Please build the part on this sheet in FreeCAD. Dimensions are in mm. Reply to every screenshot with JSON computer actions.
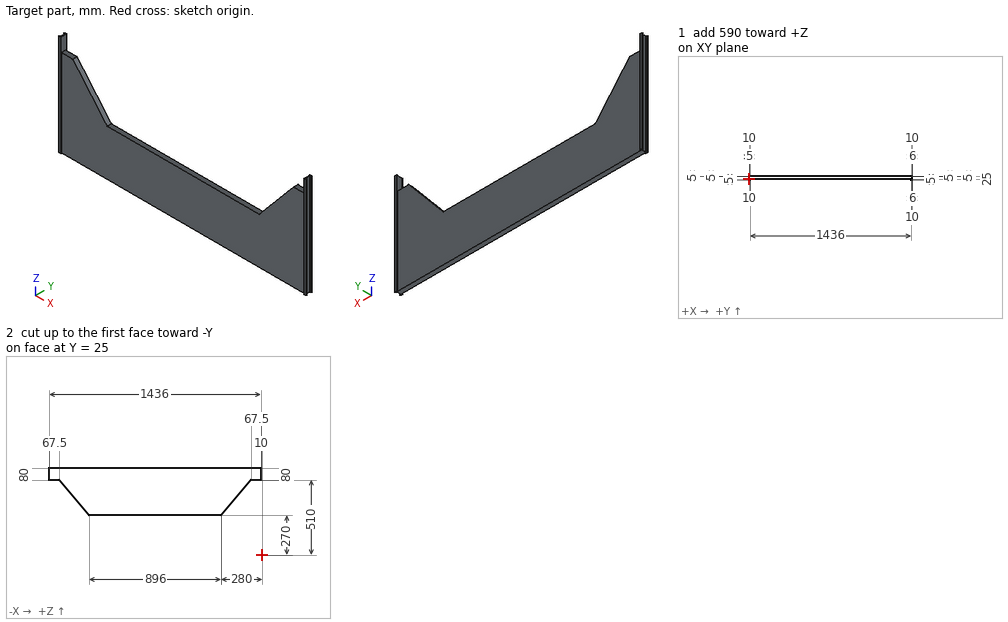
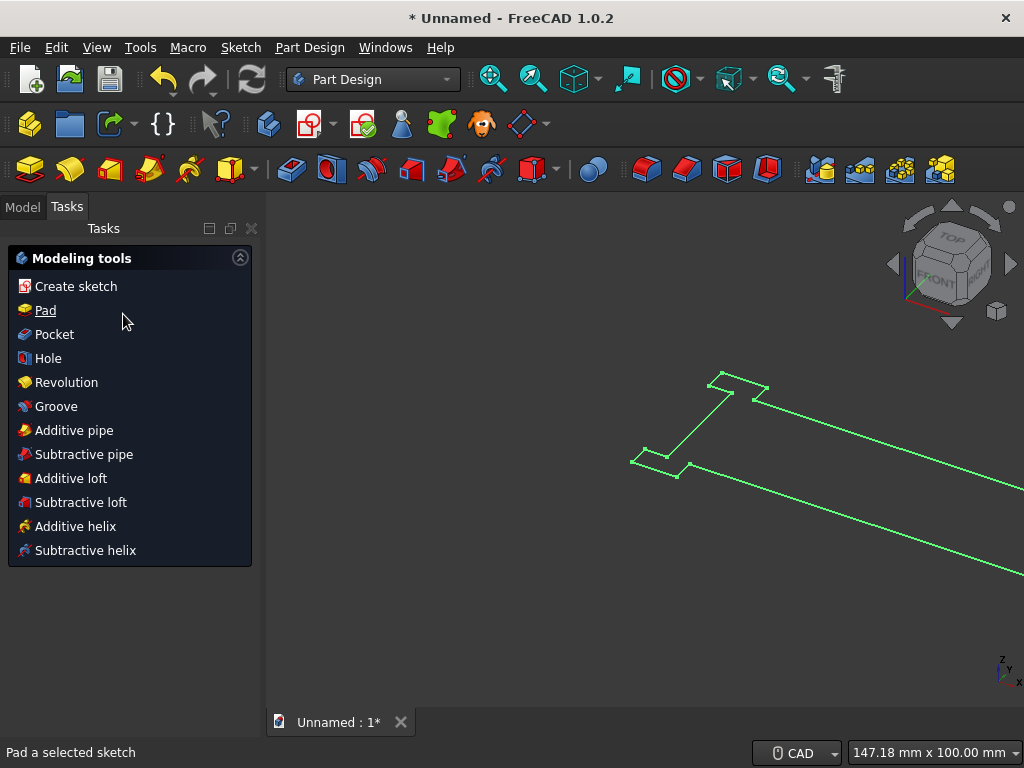
{"action": "left_click", "coordinate": [30, 170]}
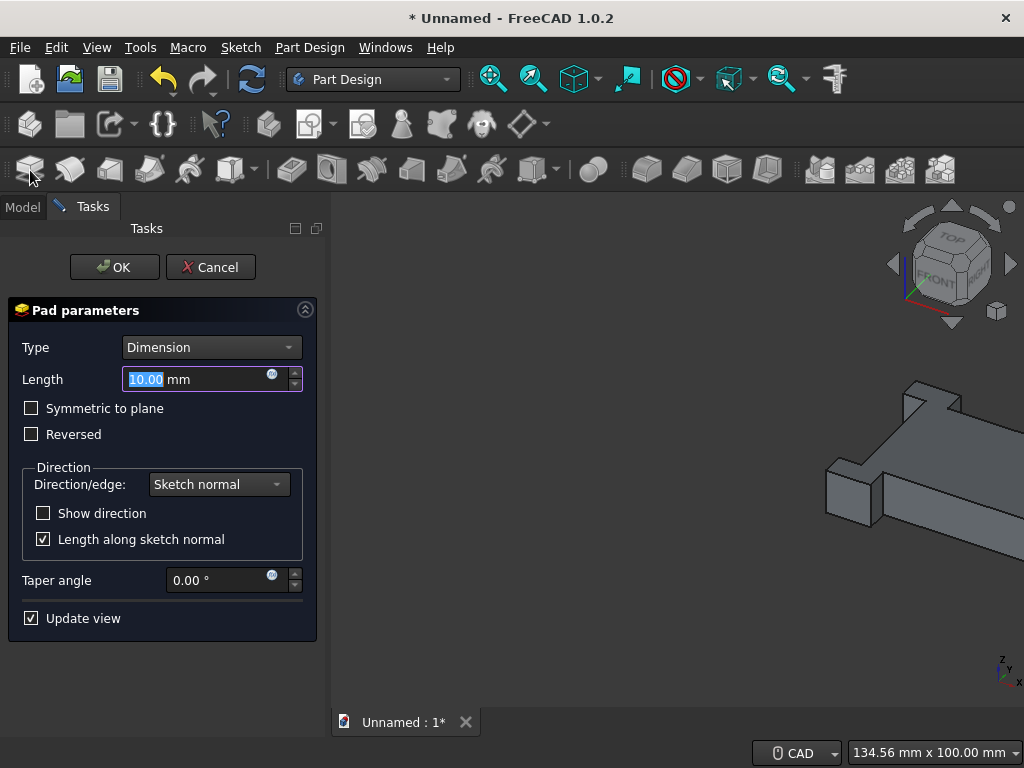
{"action": "type", "text": "590"}
{"action": "key", "text": "Tab"}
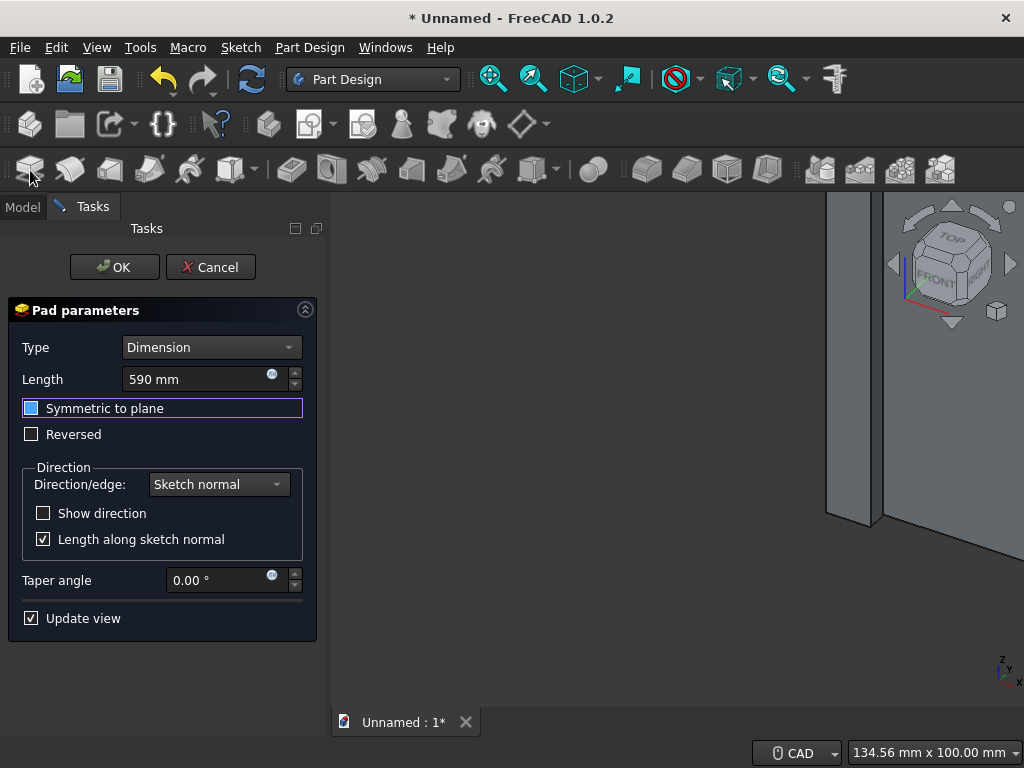
{"action": "left_click", "coordinate": [115, 267]}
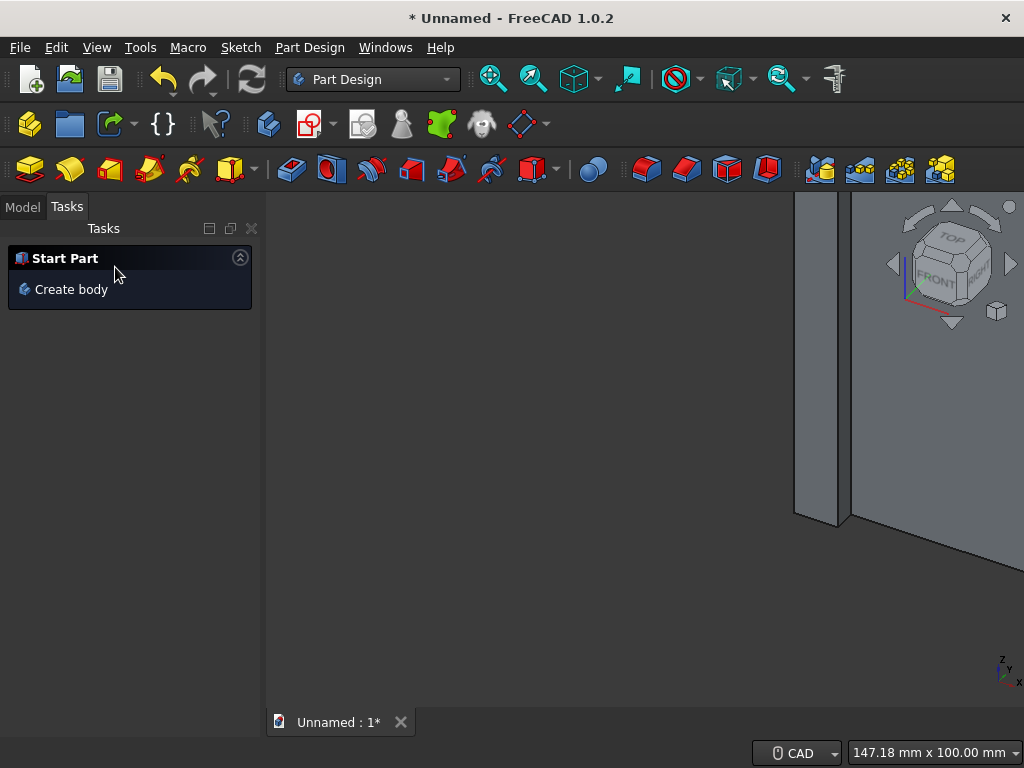
{"action": "left_click", "coordinate": [494, 80]}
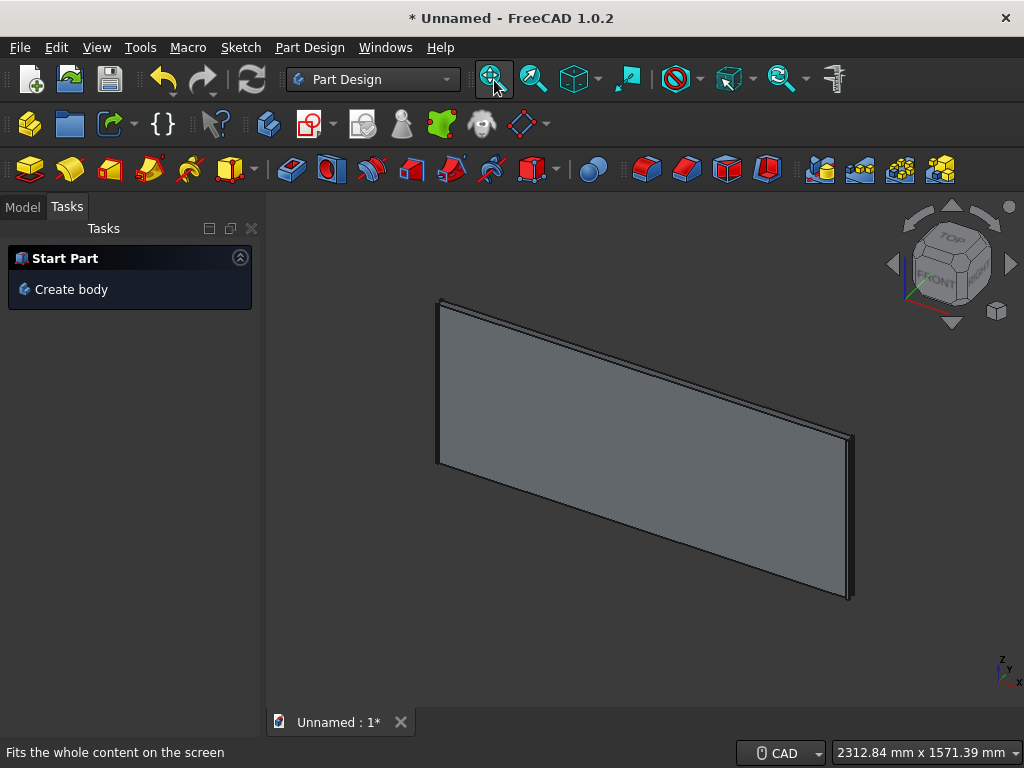
{"action": "key", "text": "4"}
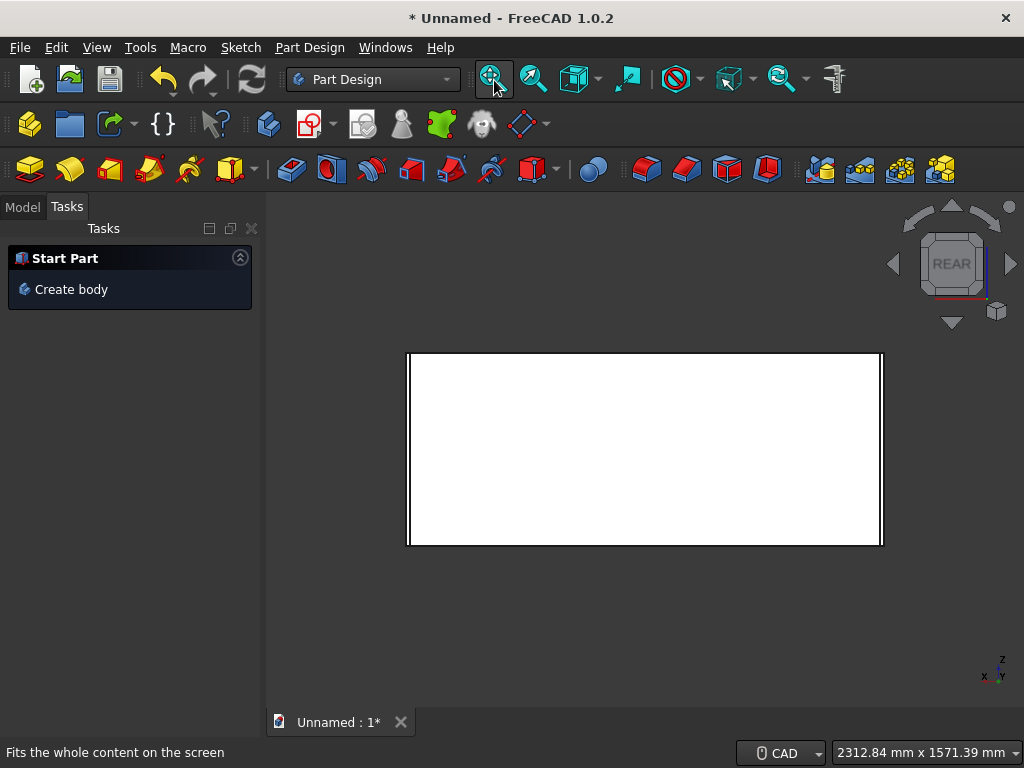
{"action": "left_click", "coordinate": [511, 448]}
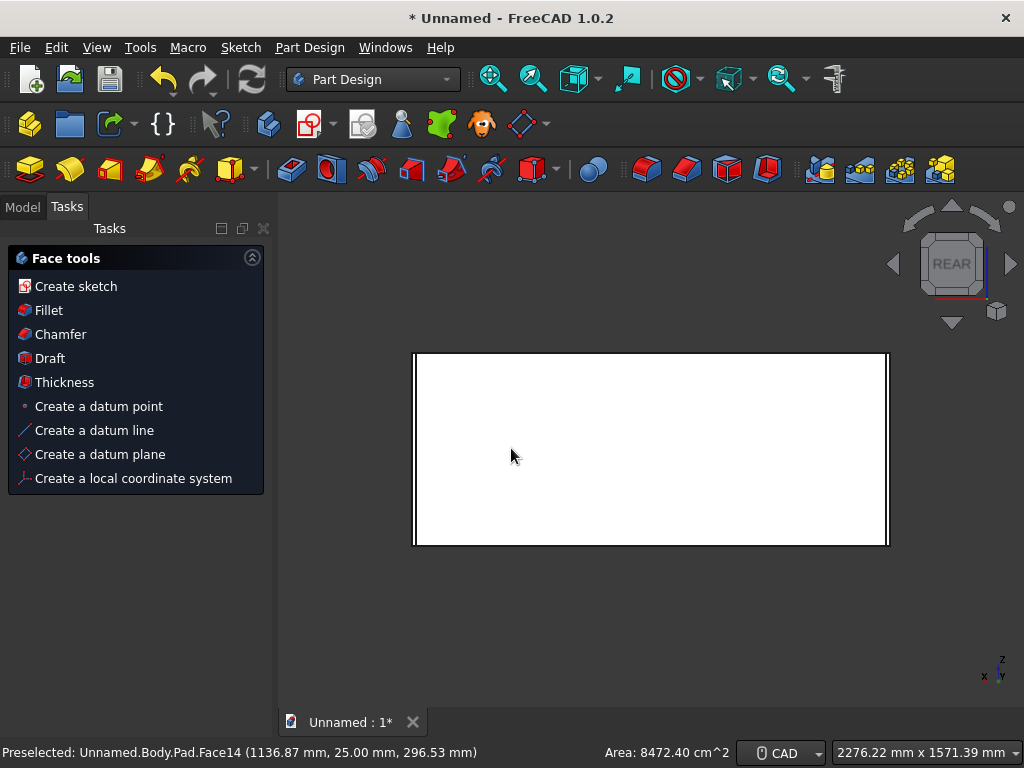
{"action": "left_click", "coordinate": [310, 124]}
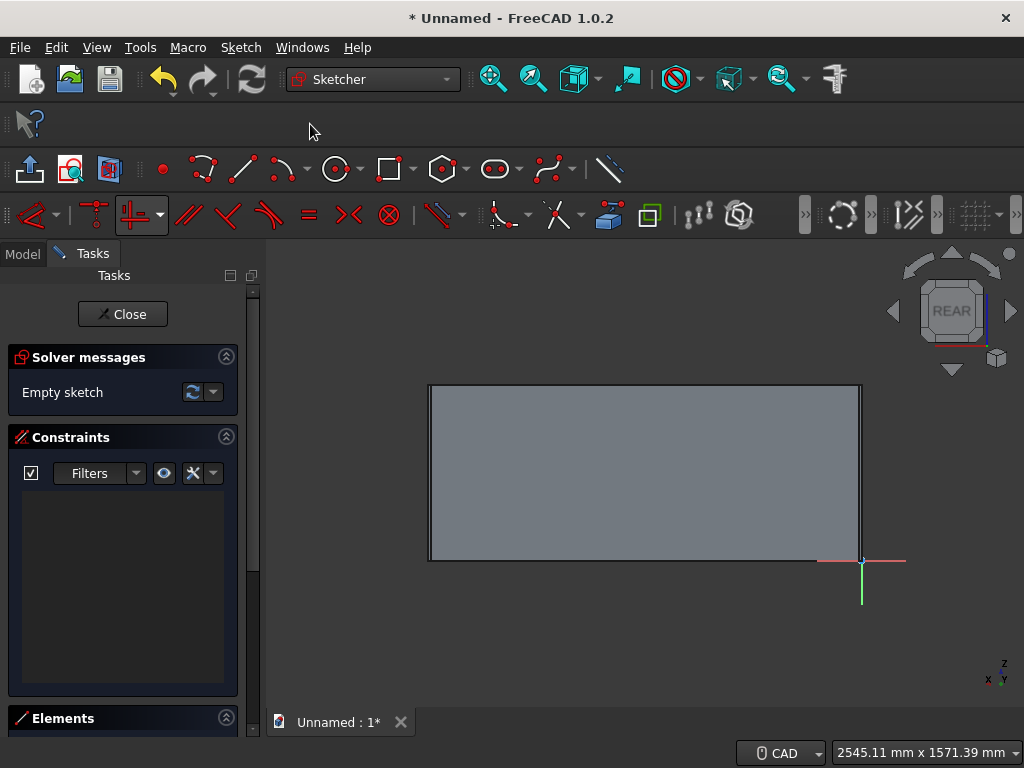
{"action": "key", "text": "q s"}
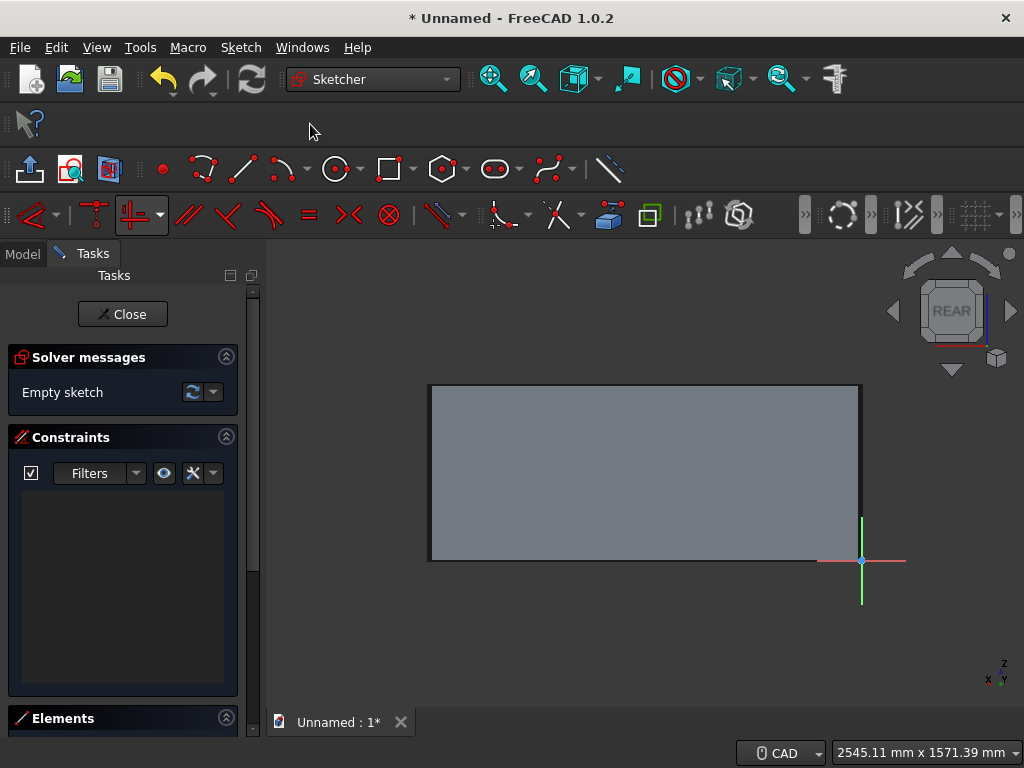
{"action": "scroll", "coordinate": [294, 473], "scroll_direction": "down", "scroll_amount": 1}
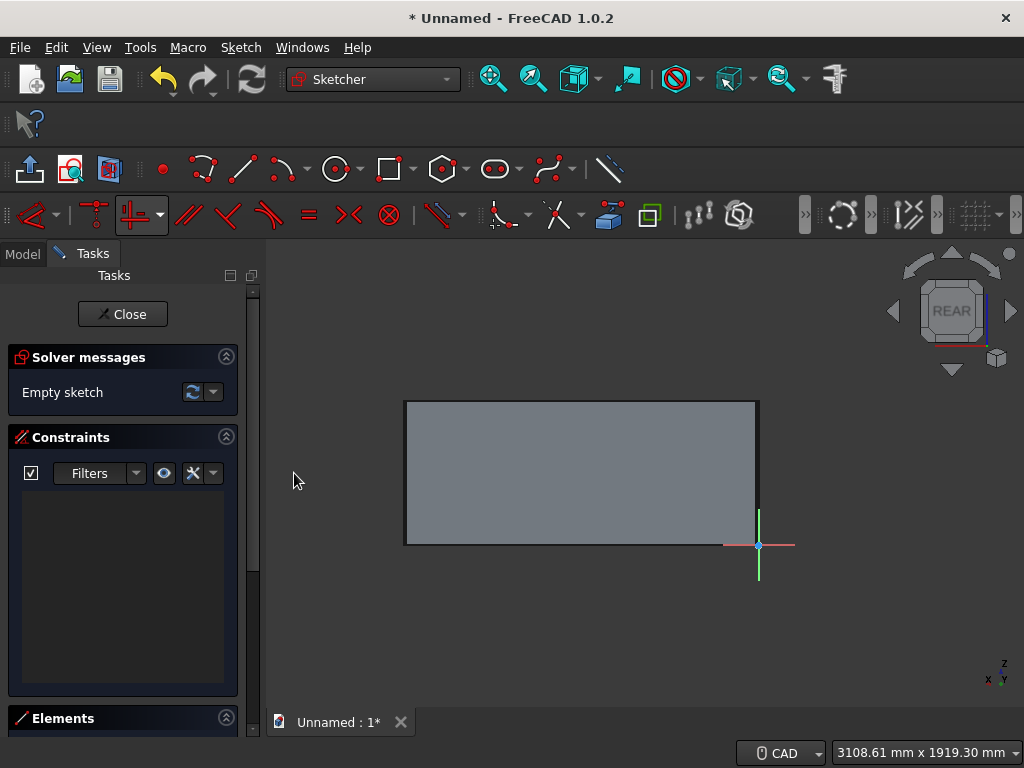
{"action": "key", "text": "g m"}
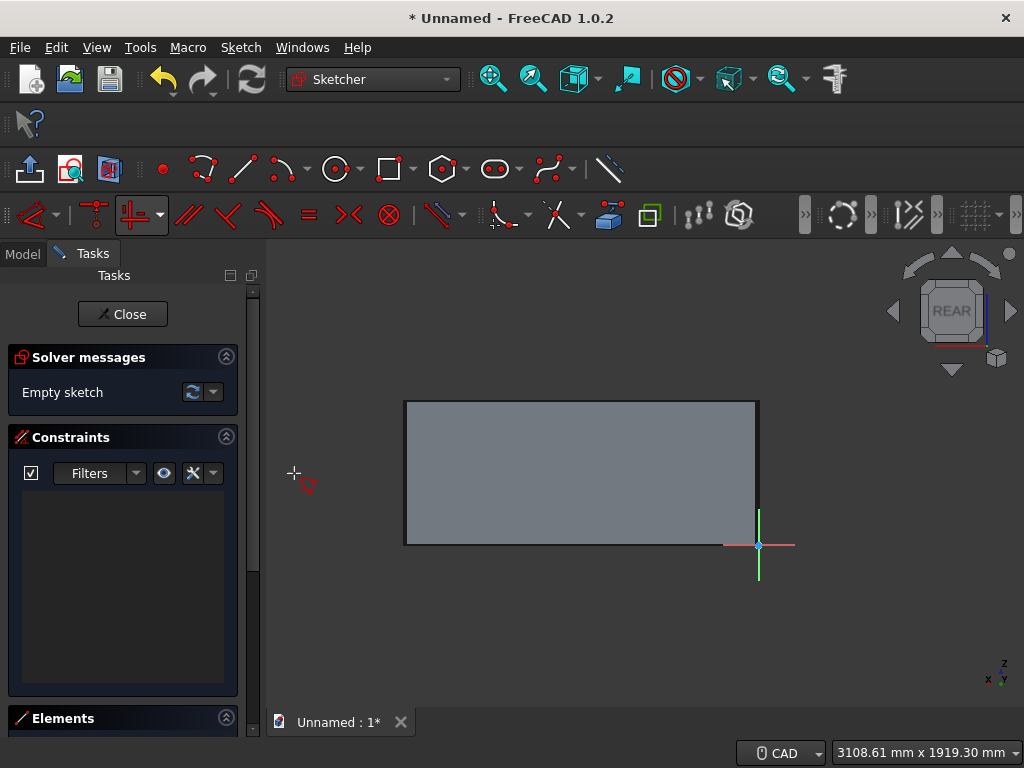
{"action": "left_click", "coordinate": [691, 479]}
{"action": "left_click", "coordinate": [740, 421]}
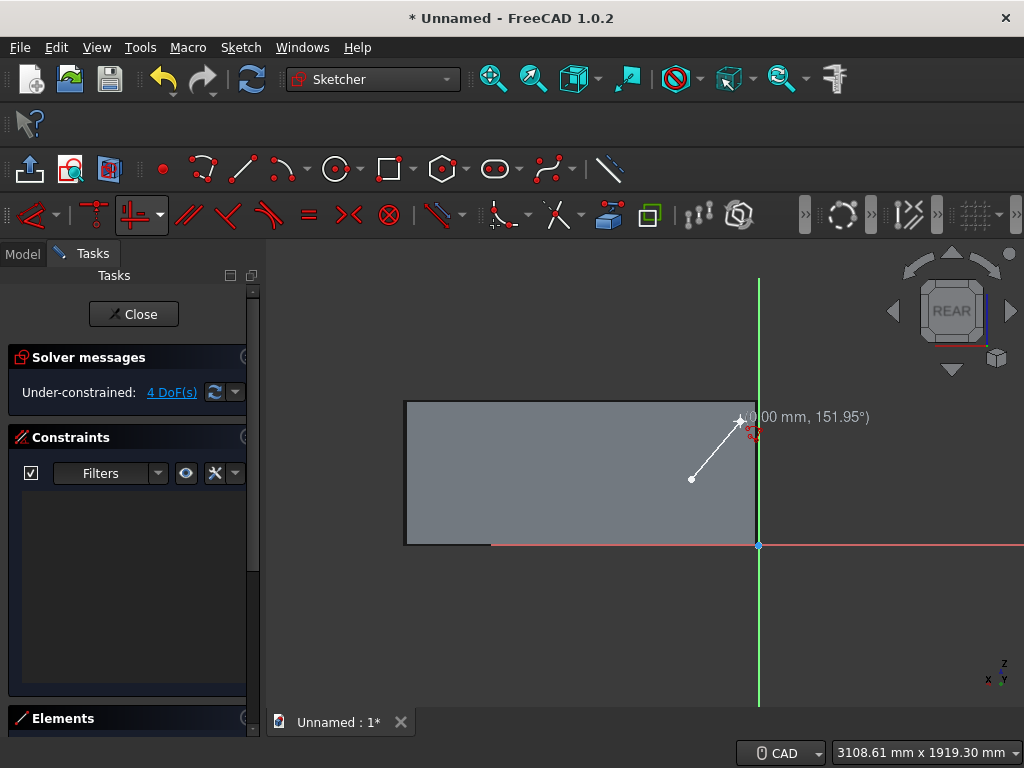
{"action": "scroll", "coordinate": [756, 421], "scroll_direction": "up", "scroll_amount": 10}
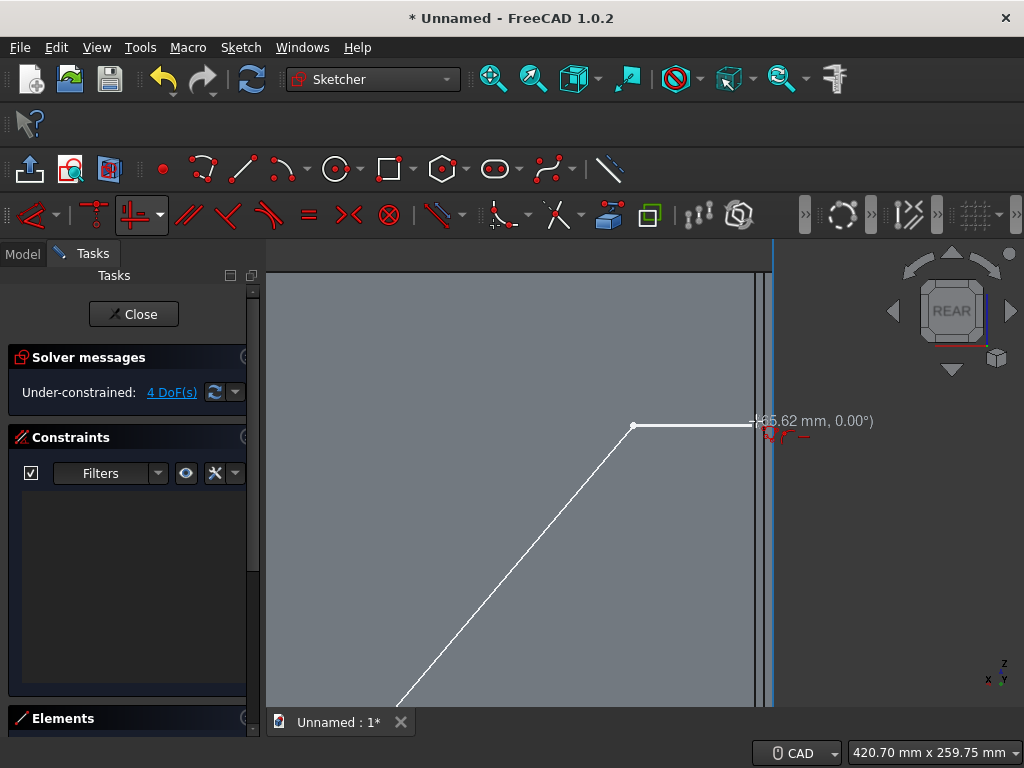
{"action": "left_click", "coordinate": [755, 419]}
{"action": "left_click", "coordinate": [755, 272]}